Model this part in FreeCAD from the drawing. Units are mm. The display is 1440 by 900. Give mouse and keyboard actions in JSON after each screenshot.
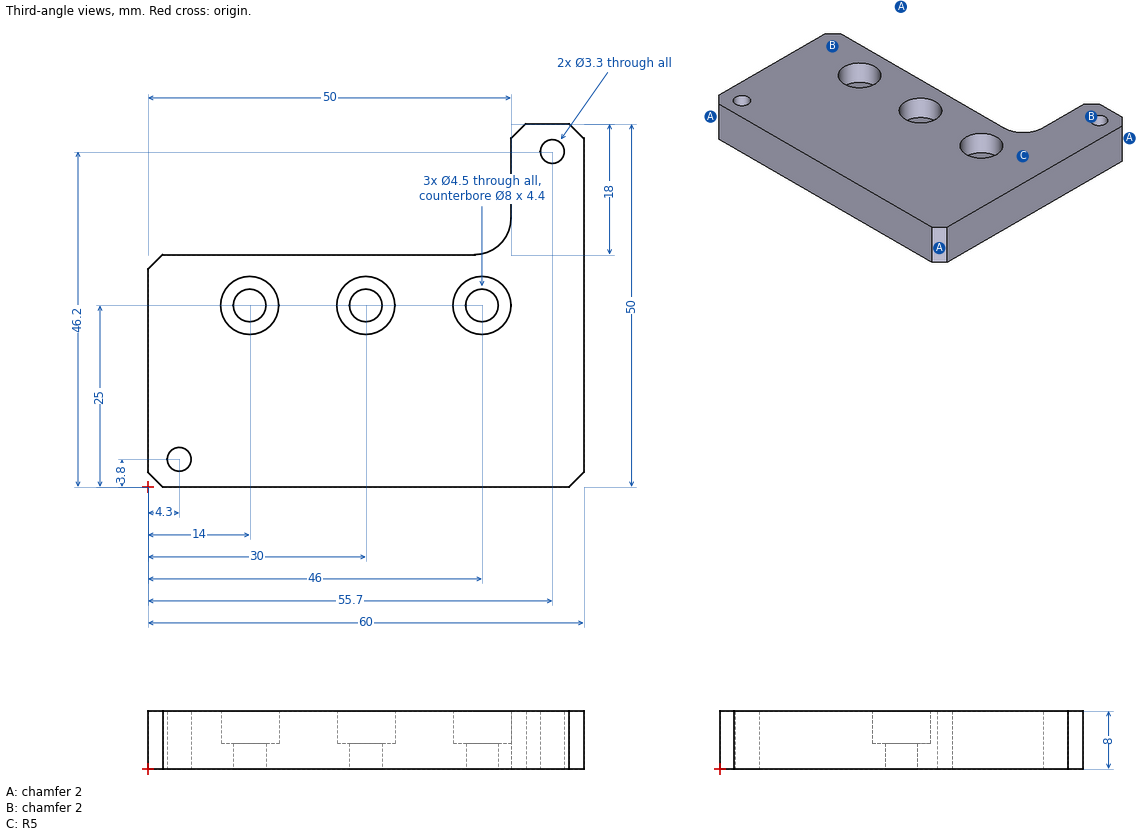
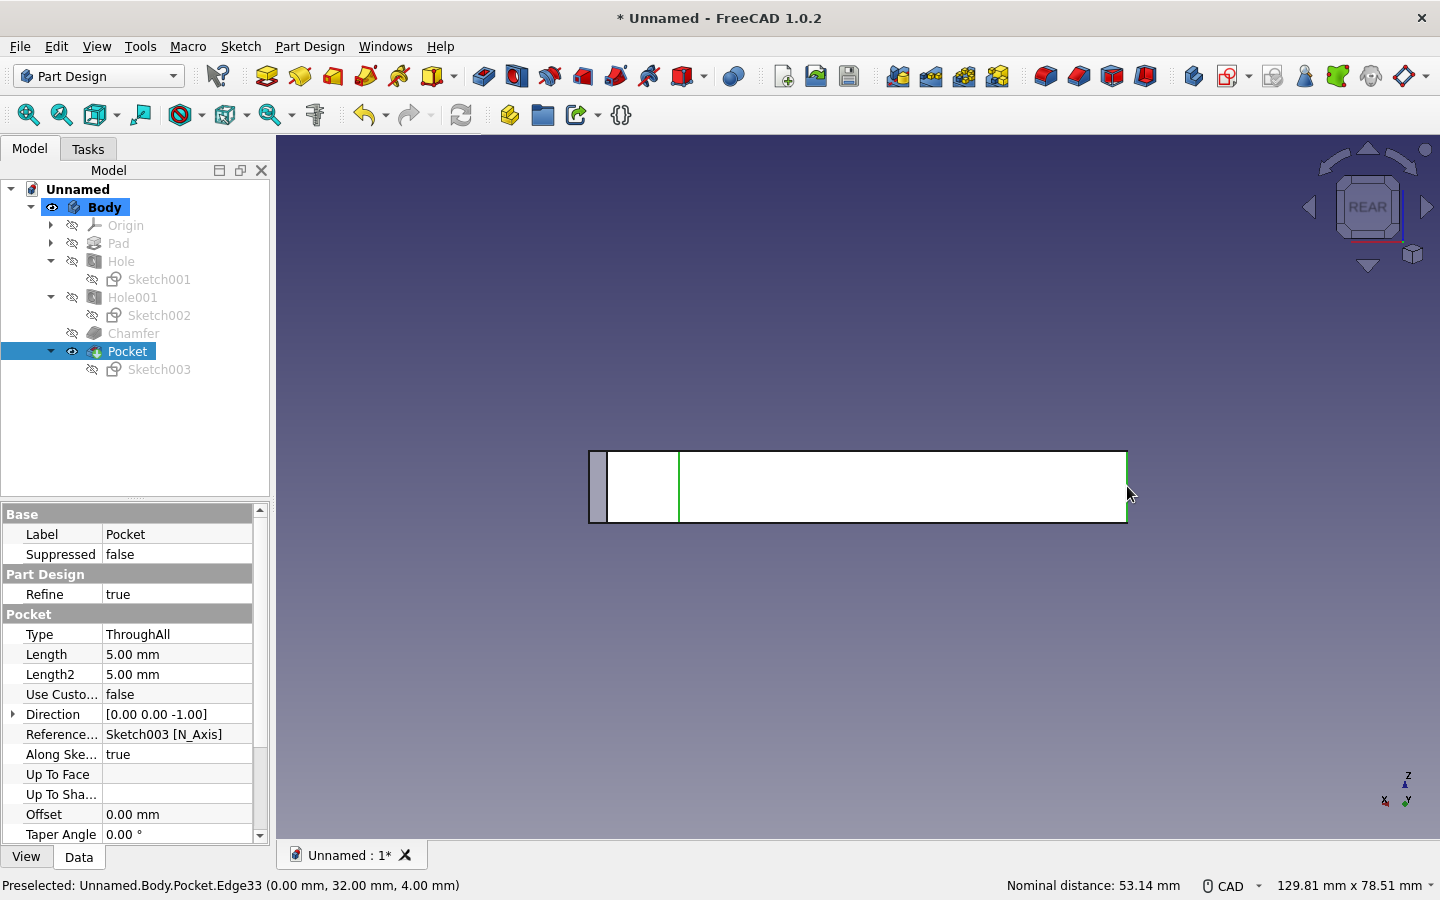
{"action": "left_click", "coordinate": [1079, 76]}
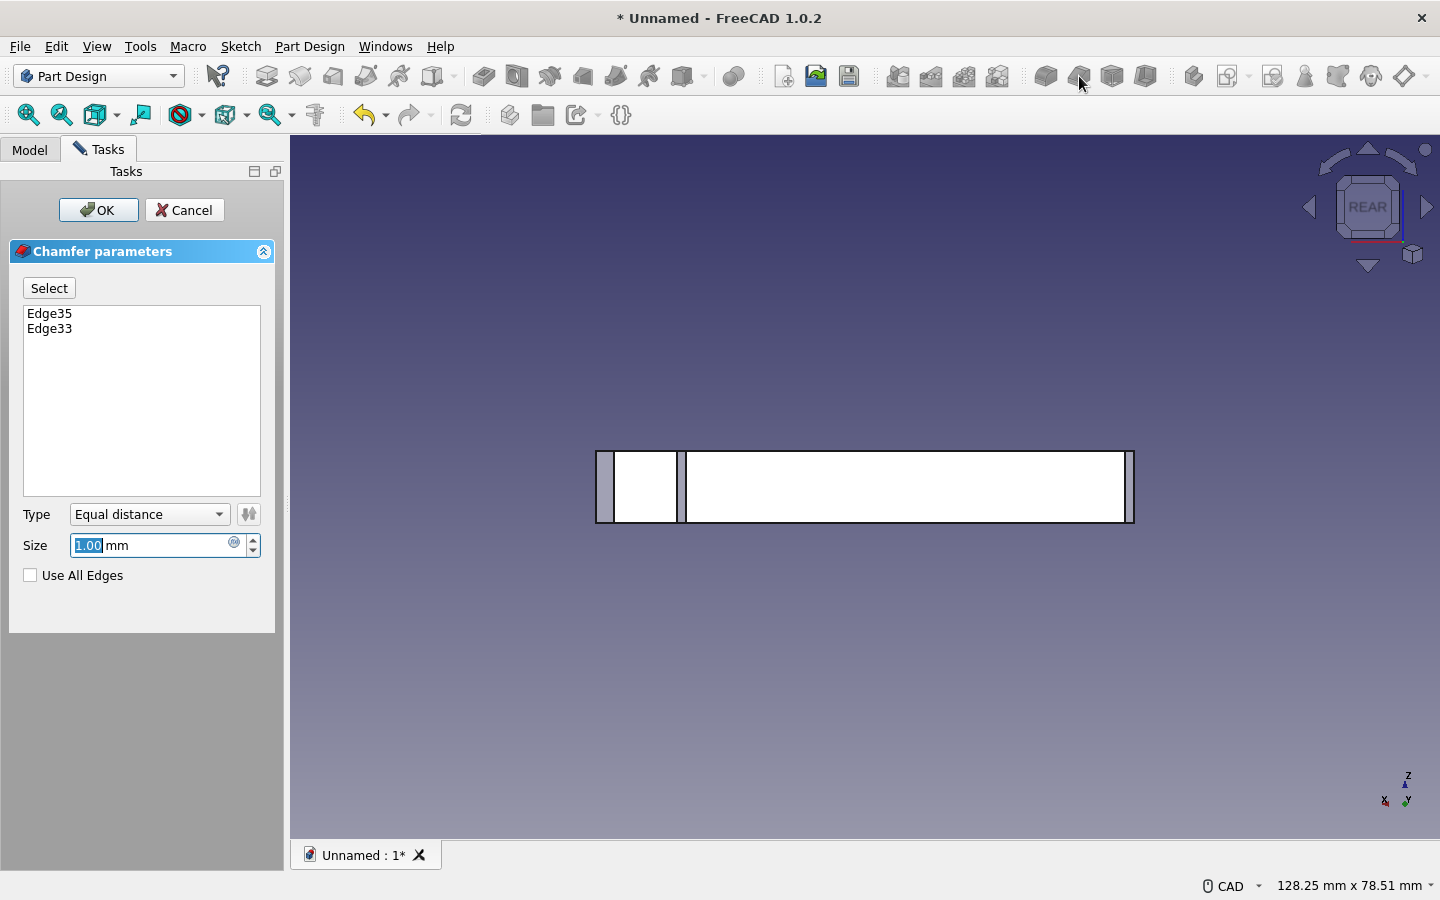
{"action": "type", "text": "2"}
{"action": "key", "text": "Tab"}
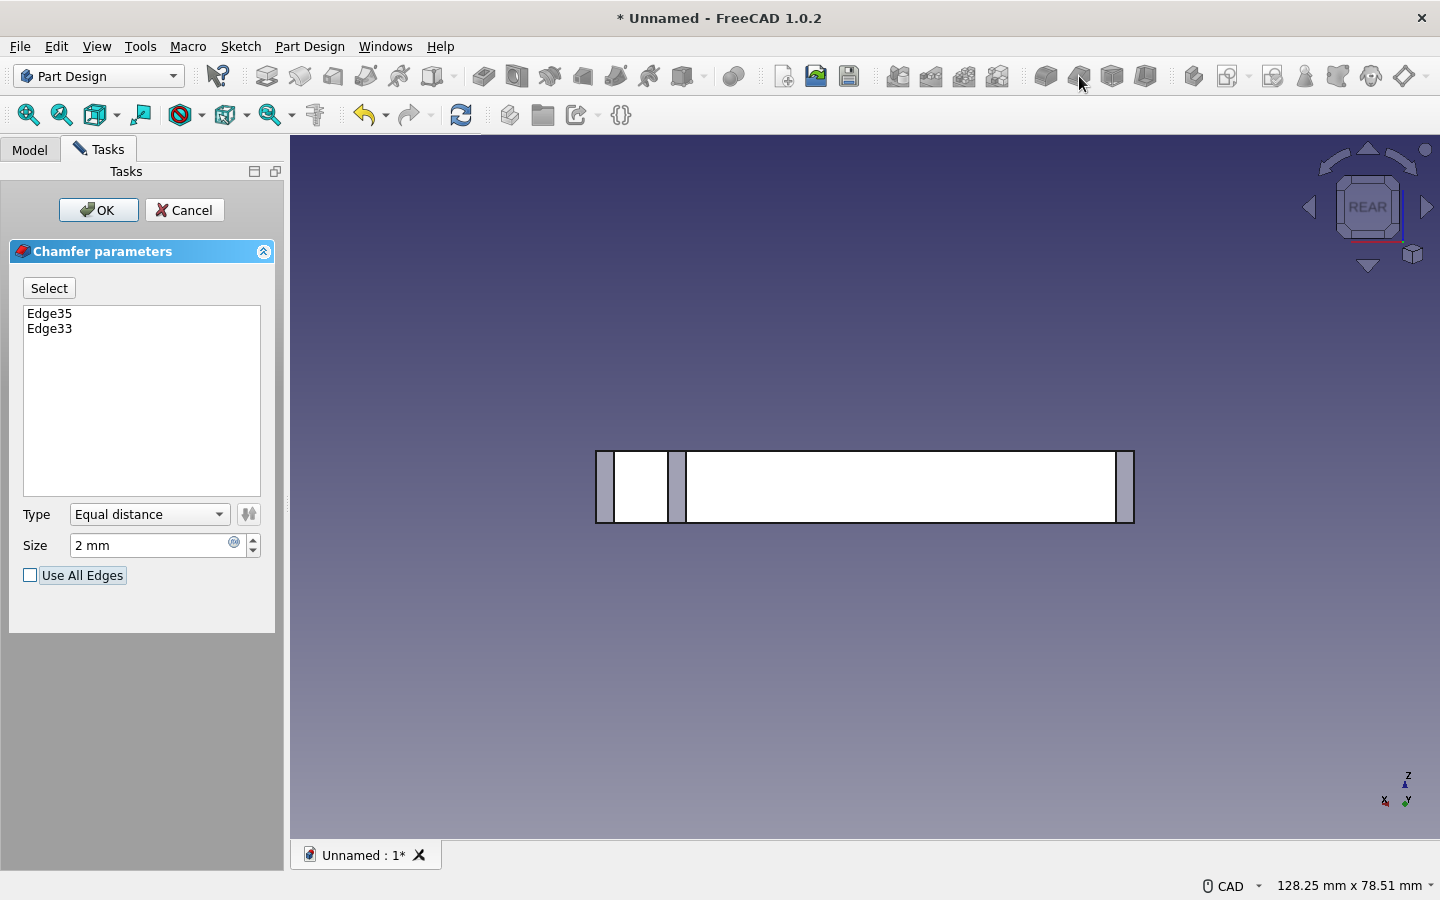
{"action": "left_click", "coordinate": [99, 210]}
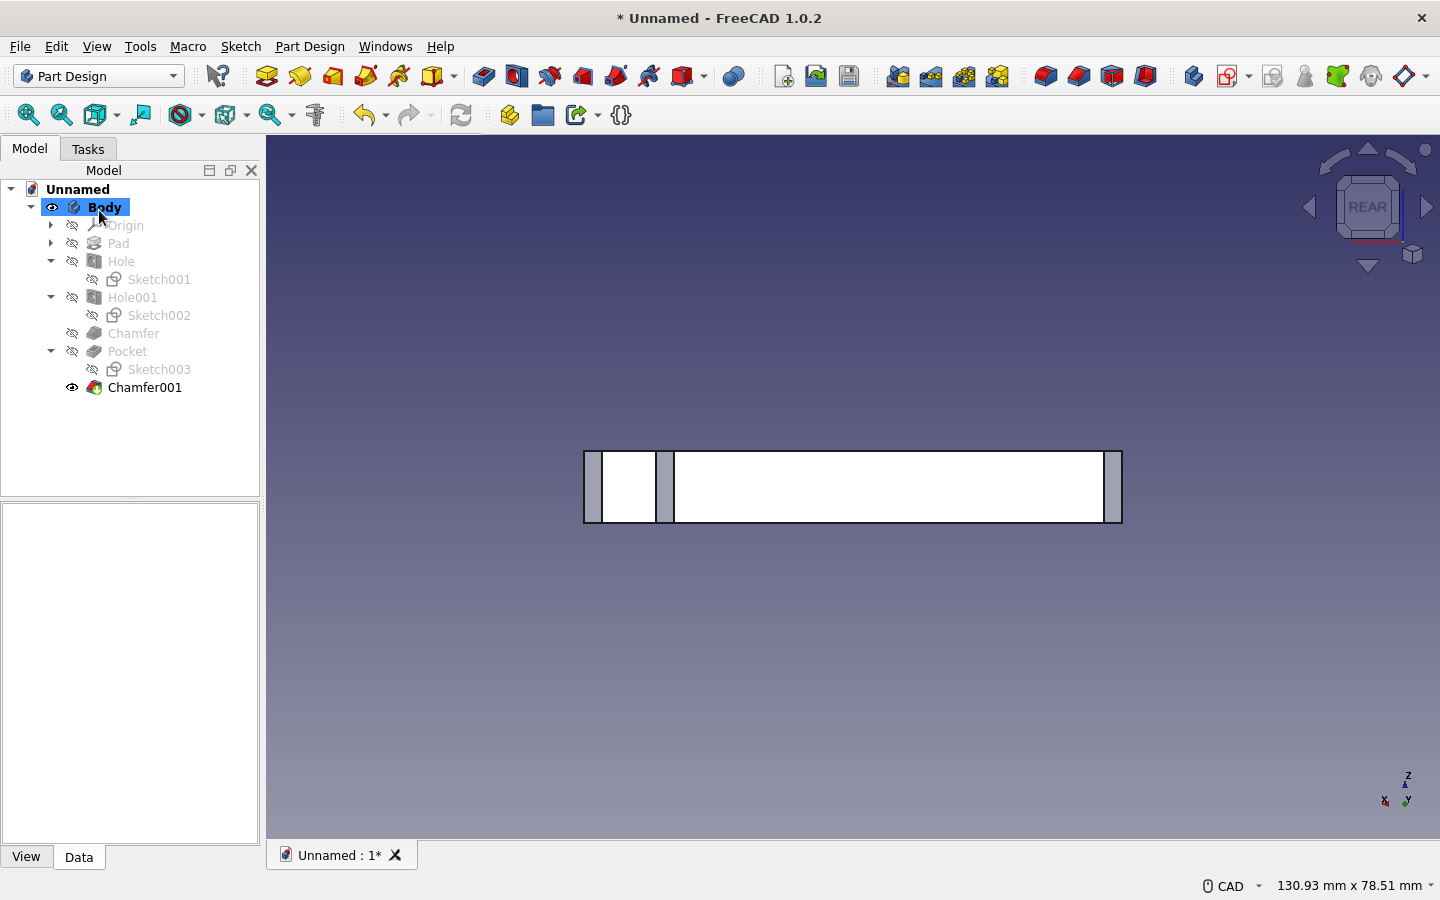
{"action": "key", "text": "0"}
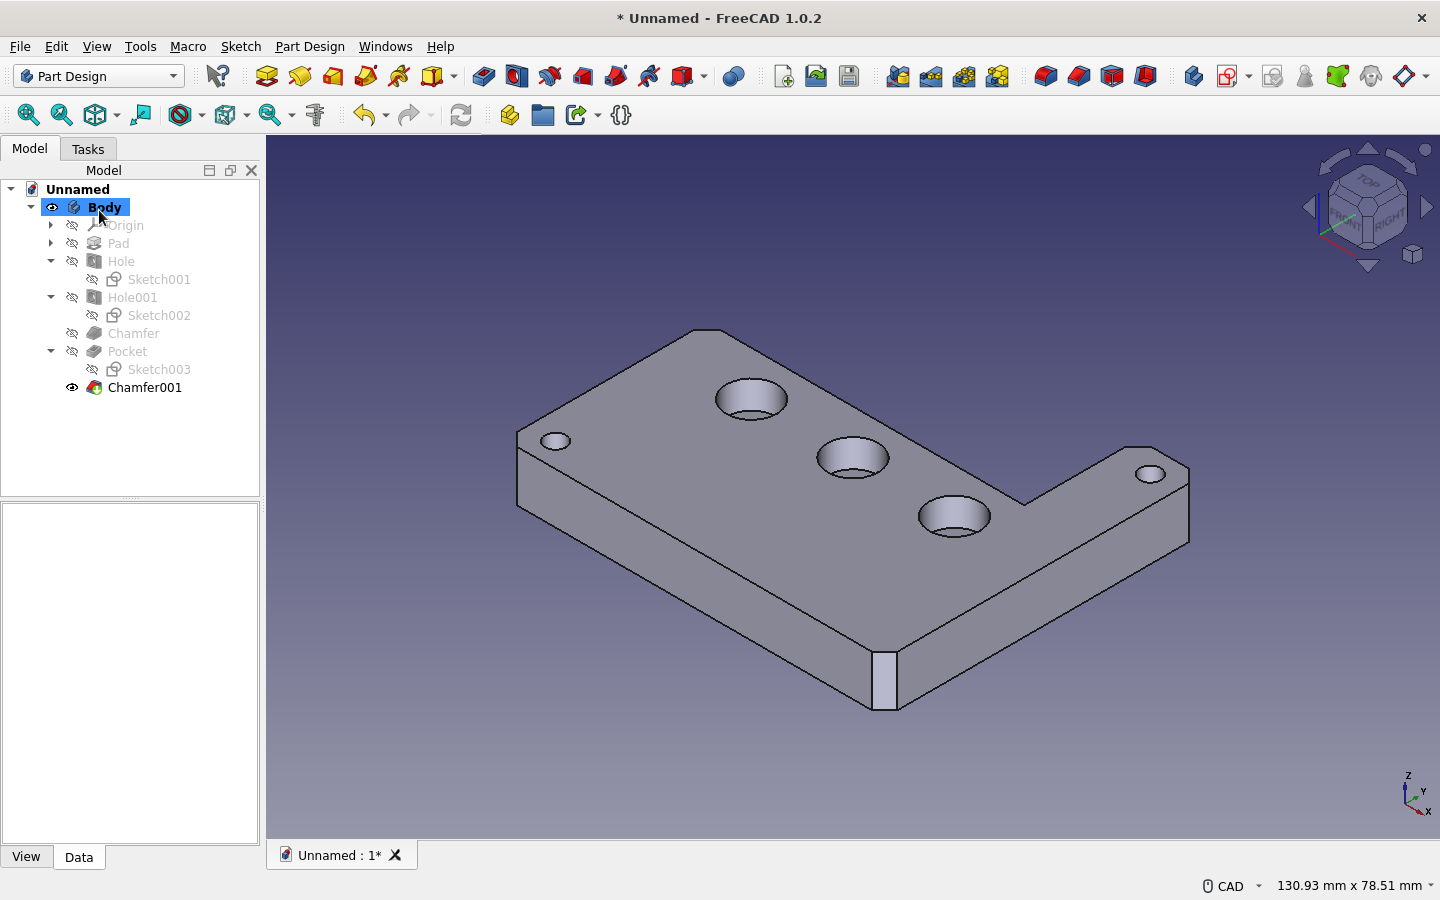
{"action": "key", "text": "2"}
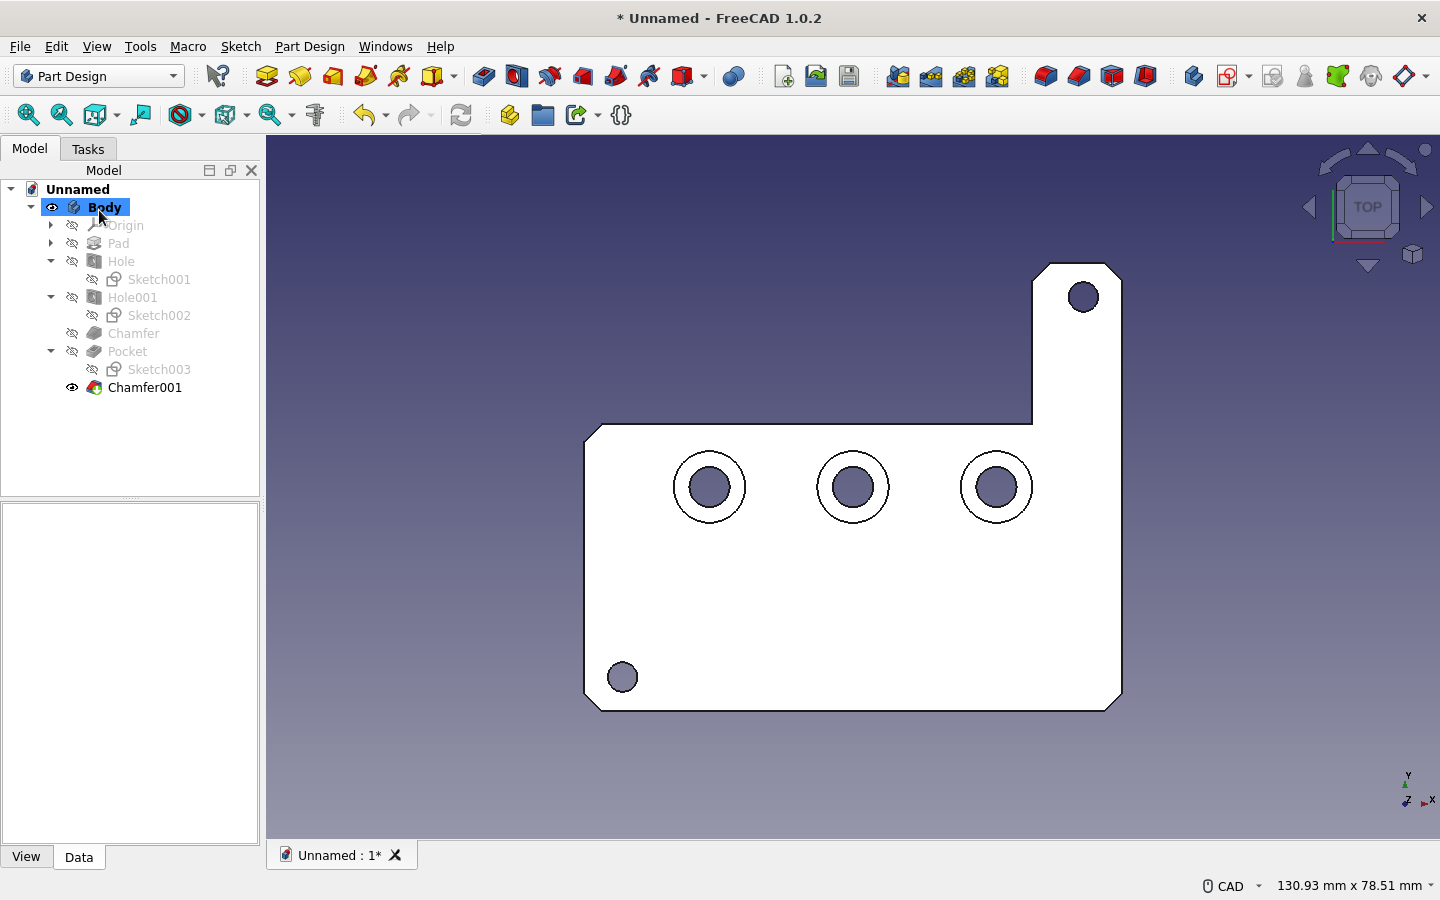
{"action": "key", "text": "1"}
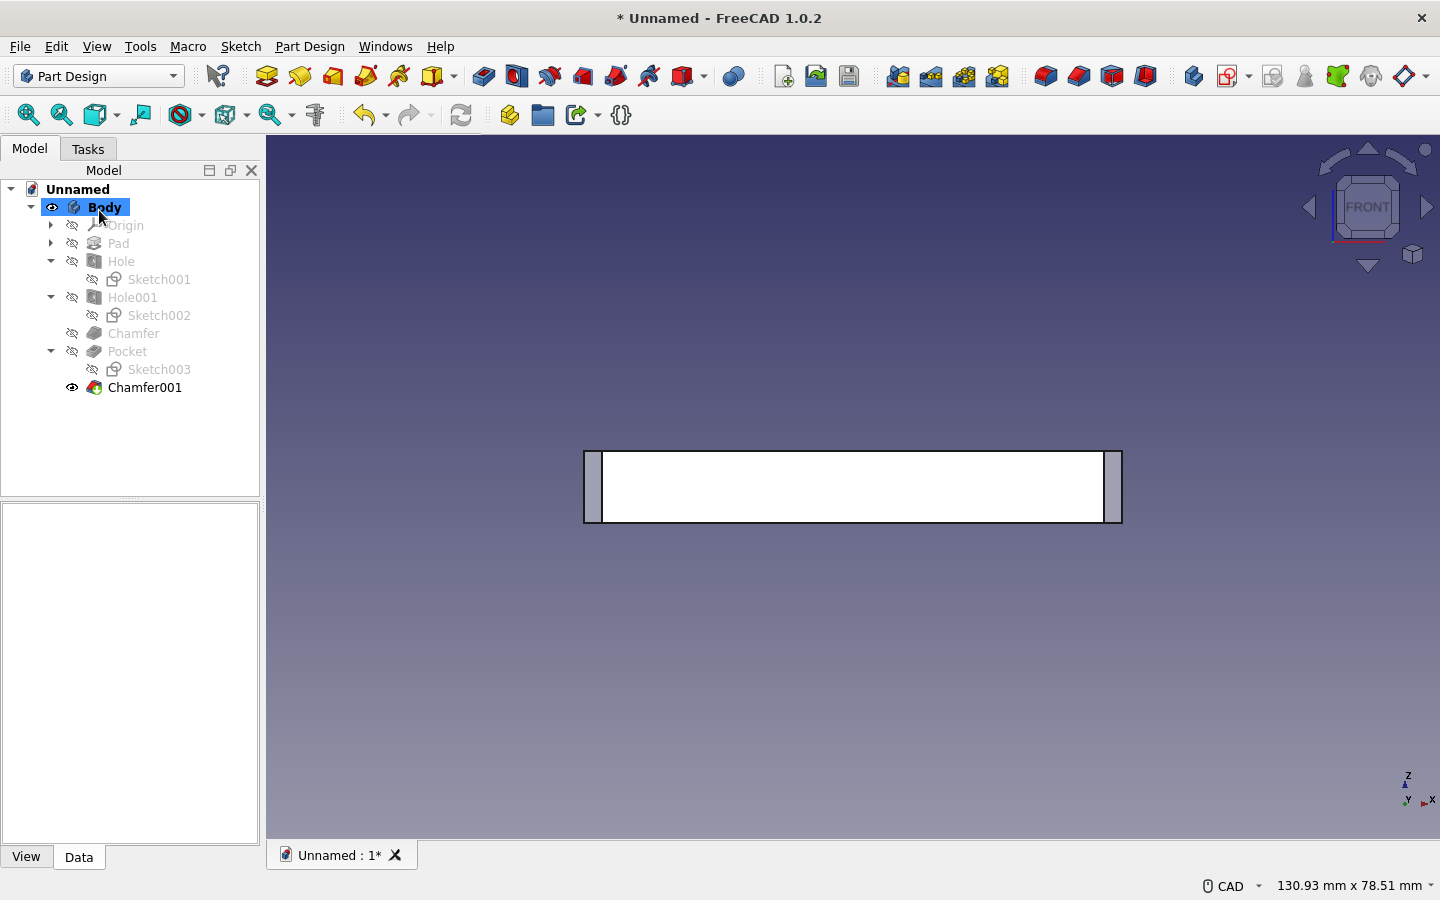
{"action": "key", "text": "3"}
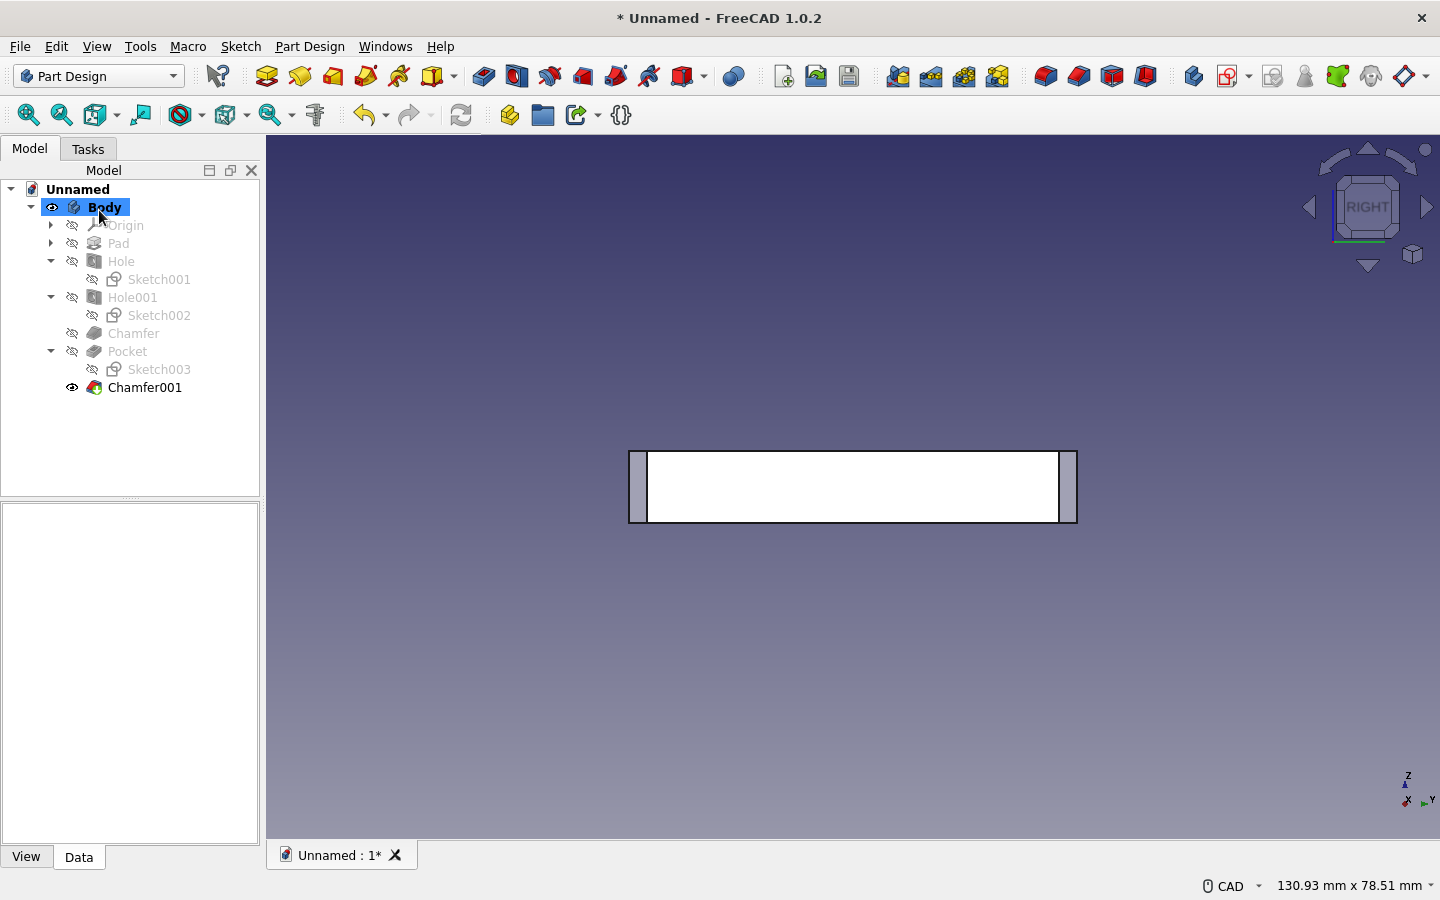
{"action": "left_click", "coordinate": [29, 116]}